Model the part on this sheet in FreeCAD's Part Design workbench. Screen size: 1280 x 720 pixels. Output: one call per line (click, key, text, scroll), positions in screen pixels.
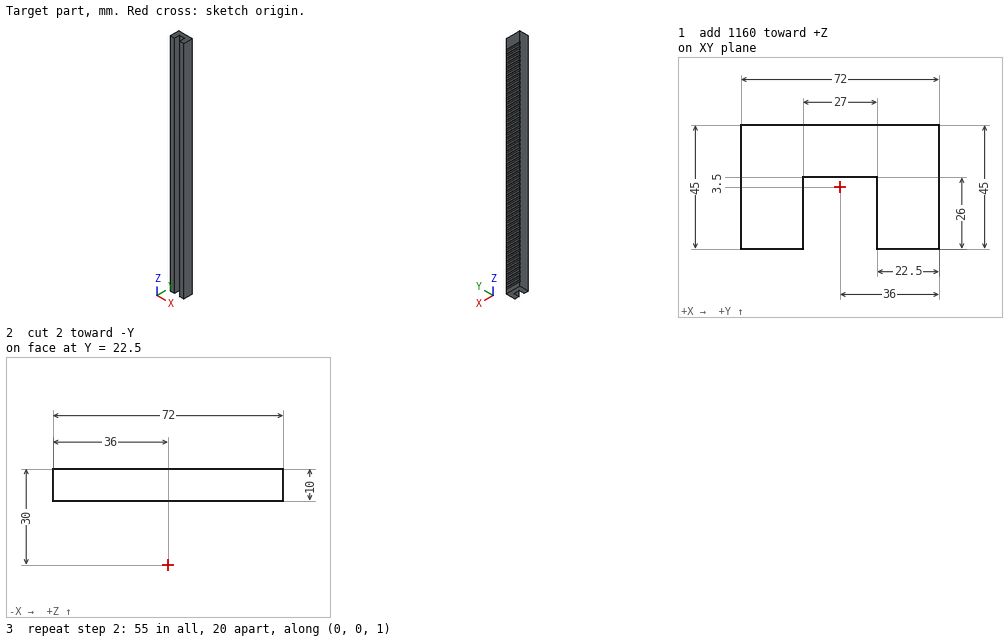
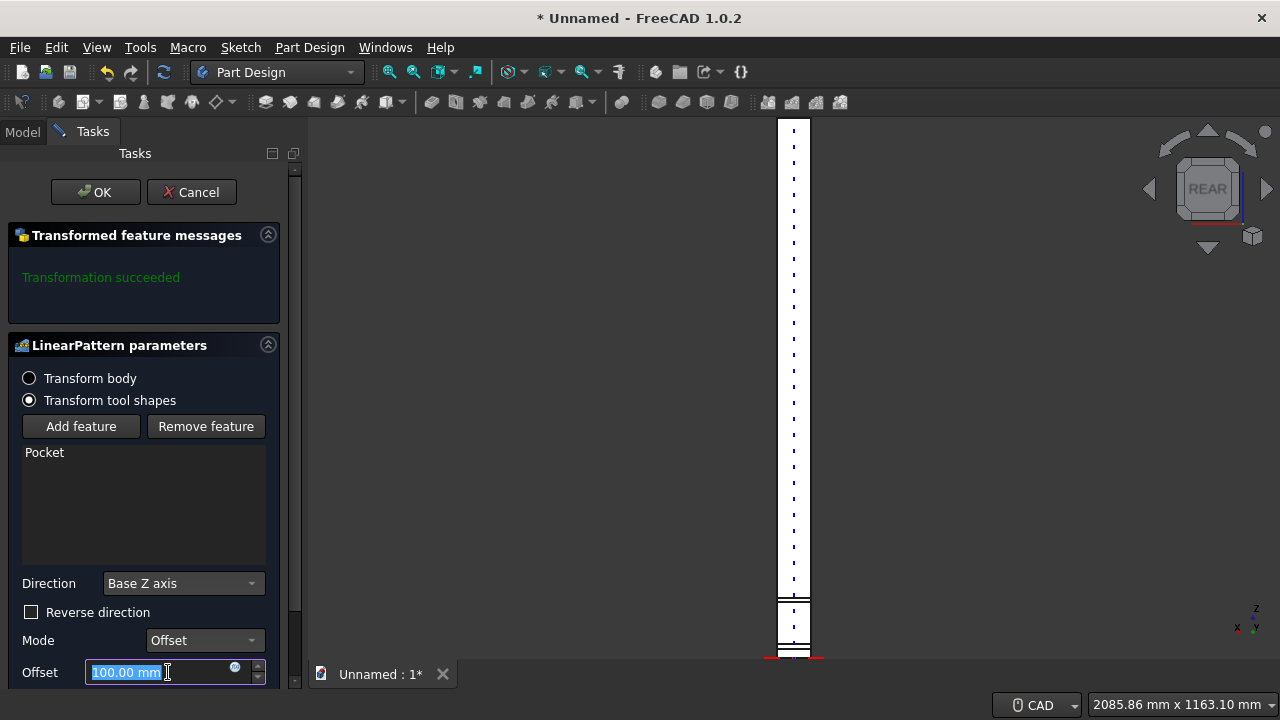
text(20)
key(Tab)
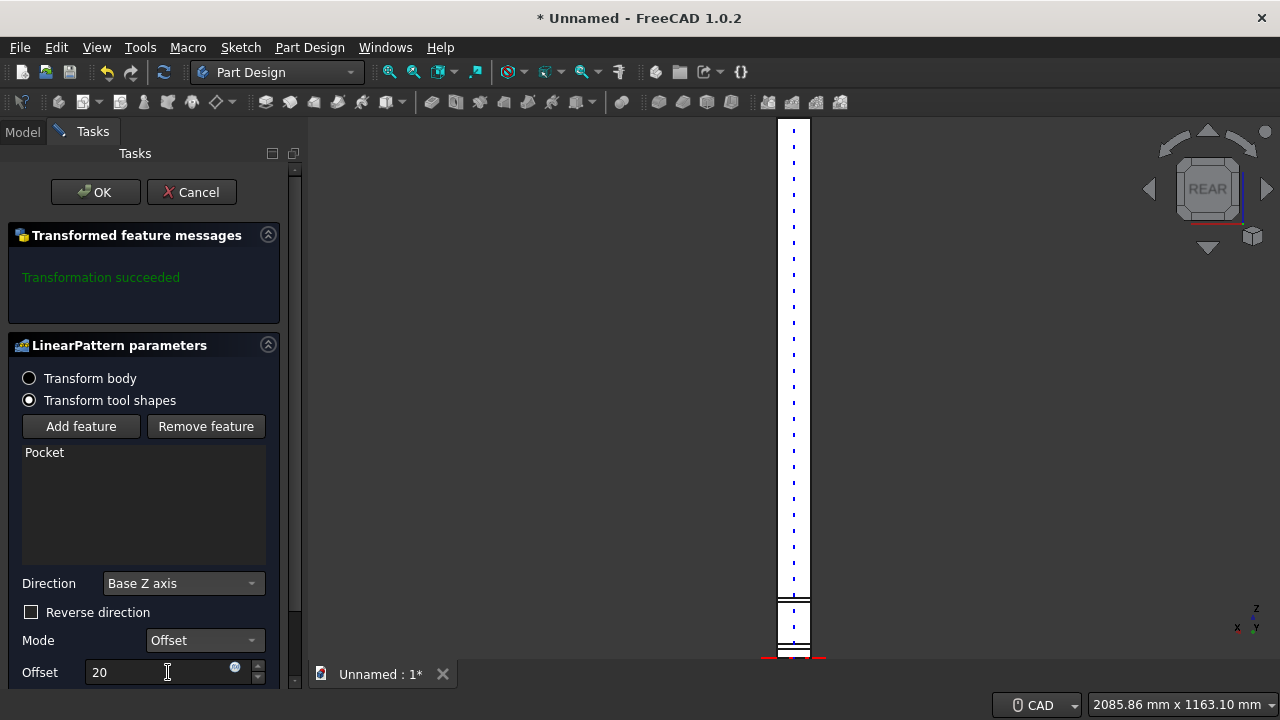
scroll(295, 426, down, 2)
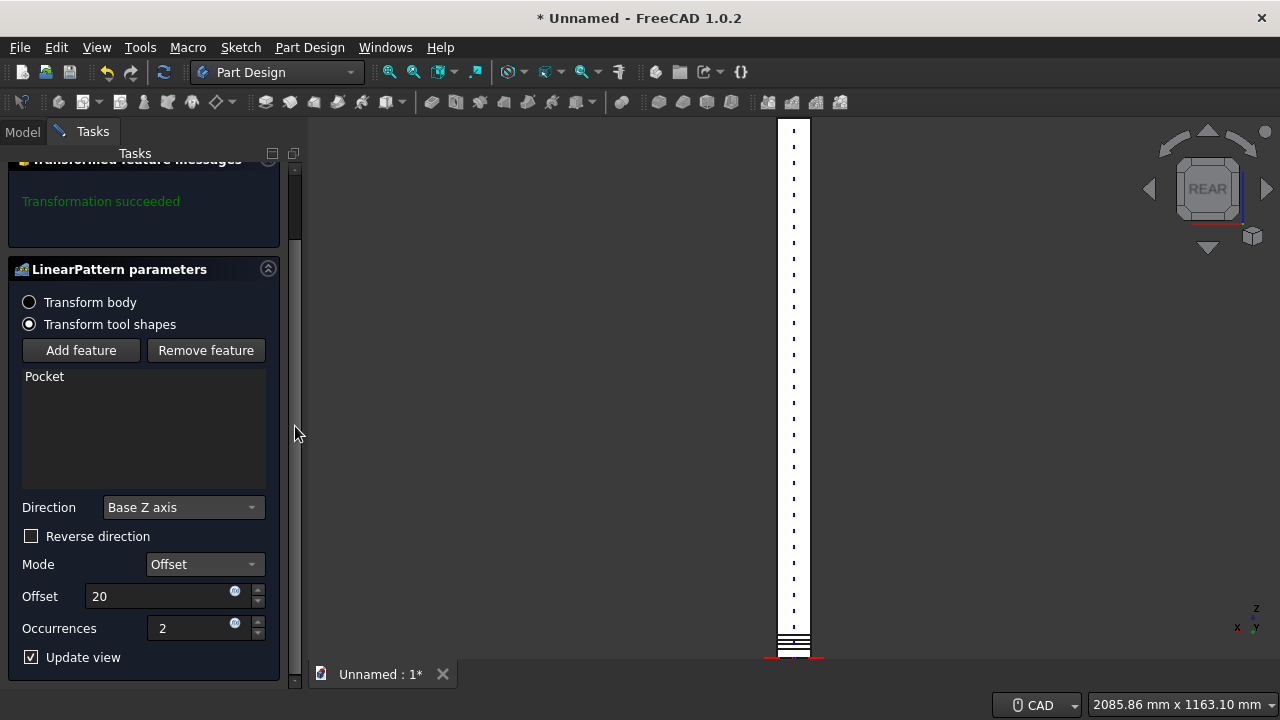
triple_click(198, 628)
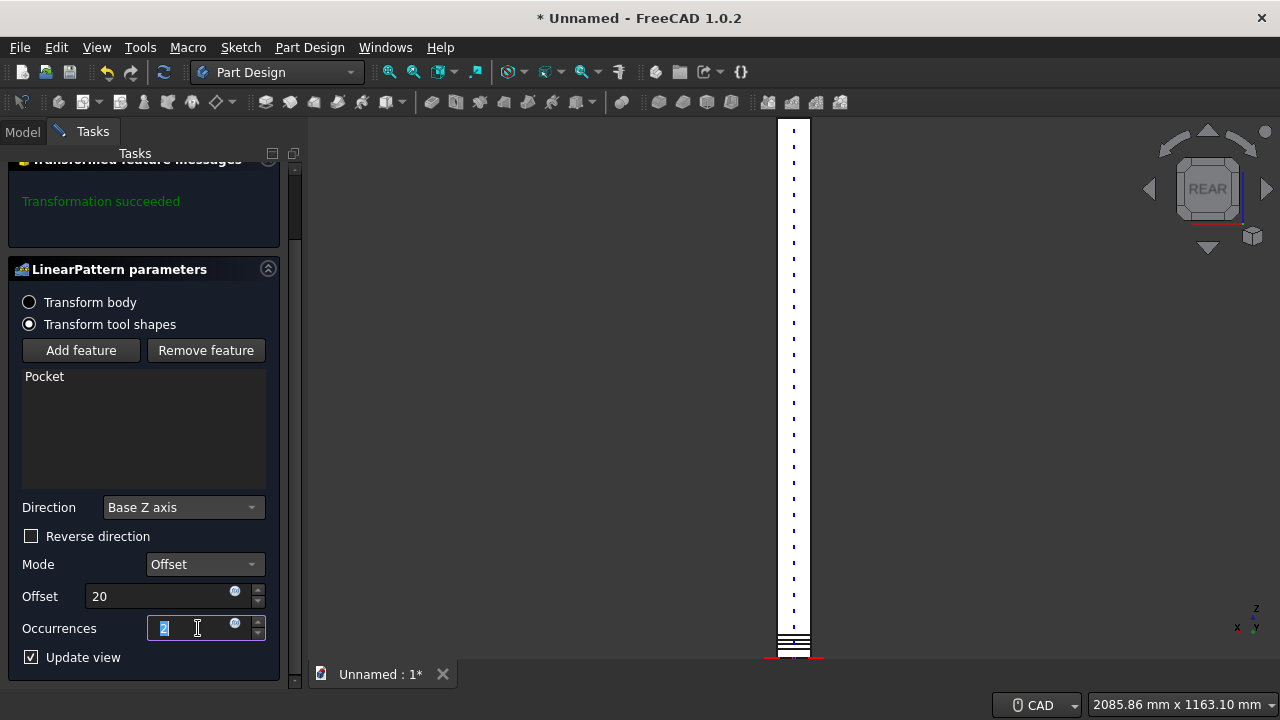
text(55)
key(Tab)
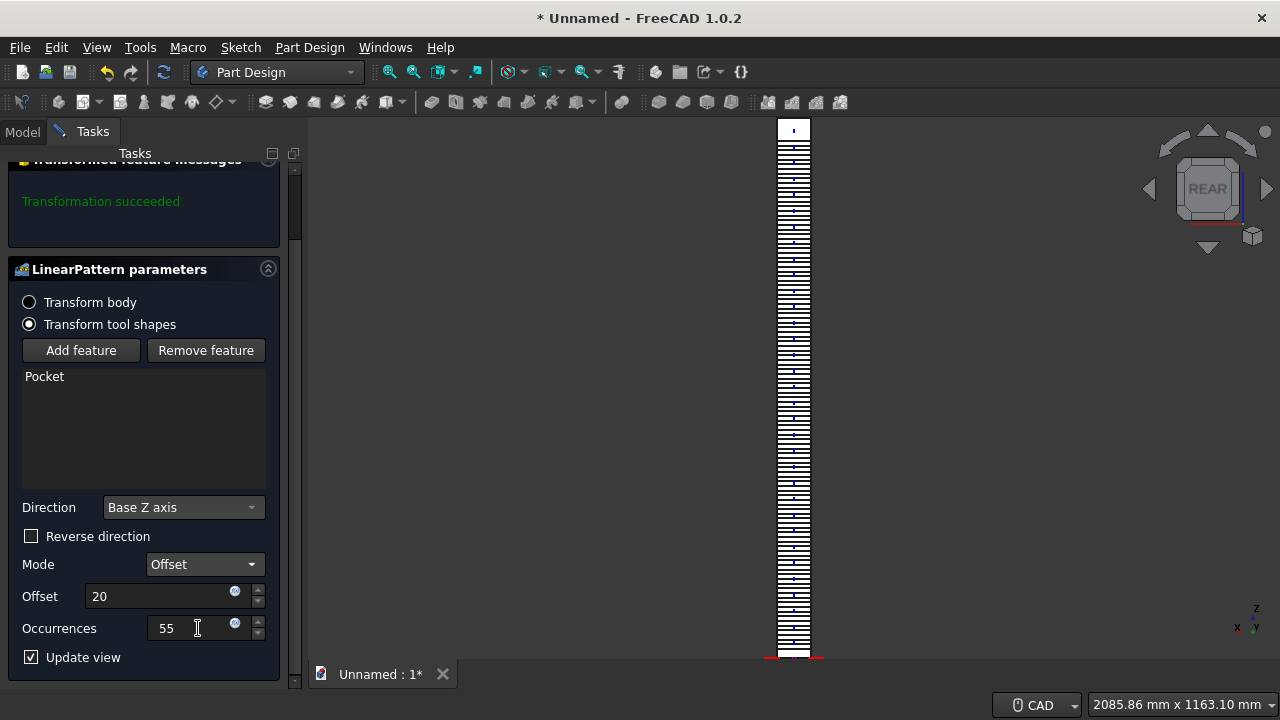
scroll(295, 426, up, 3)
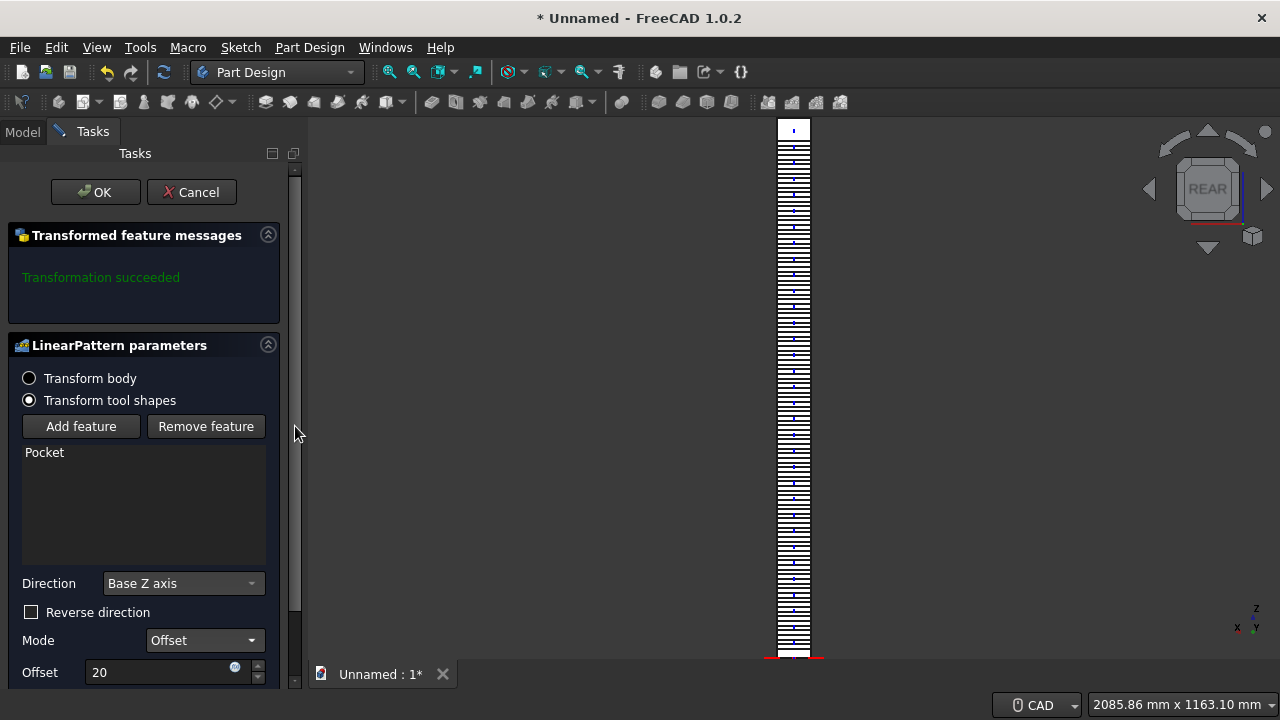
click(96, 192)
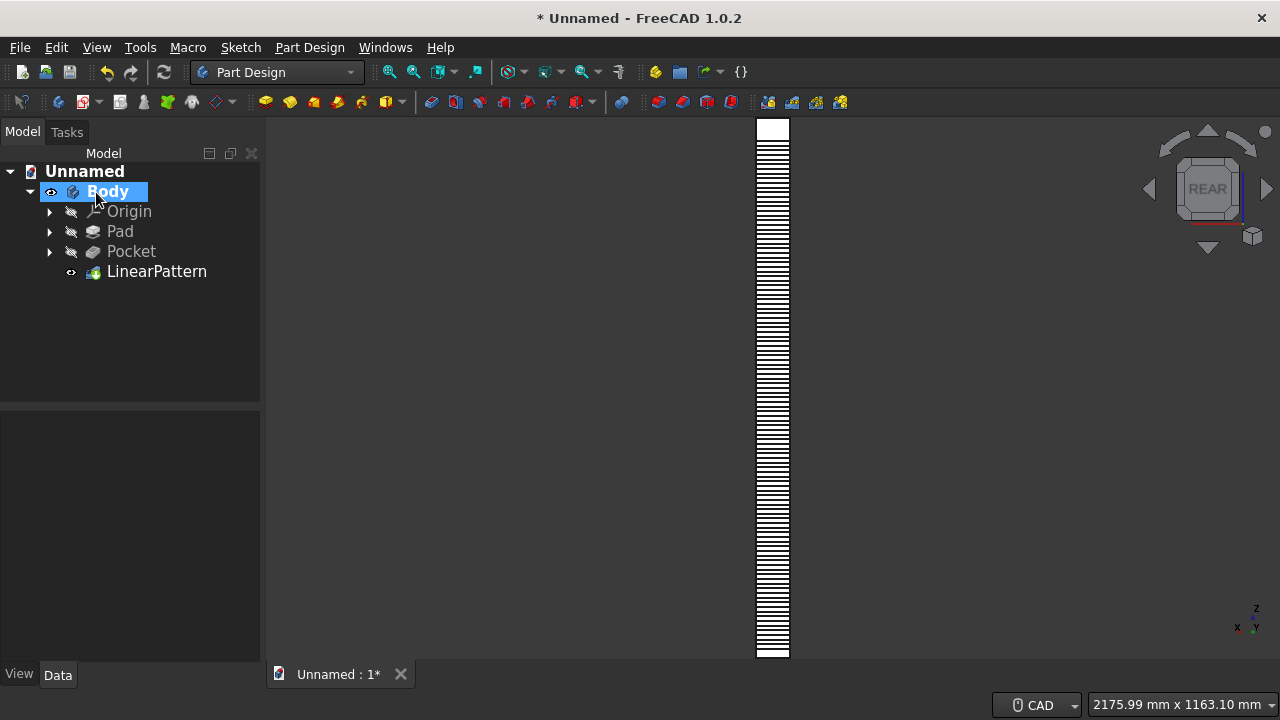
key(0)